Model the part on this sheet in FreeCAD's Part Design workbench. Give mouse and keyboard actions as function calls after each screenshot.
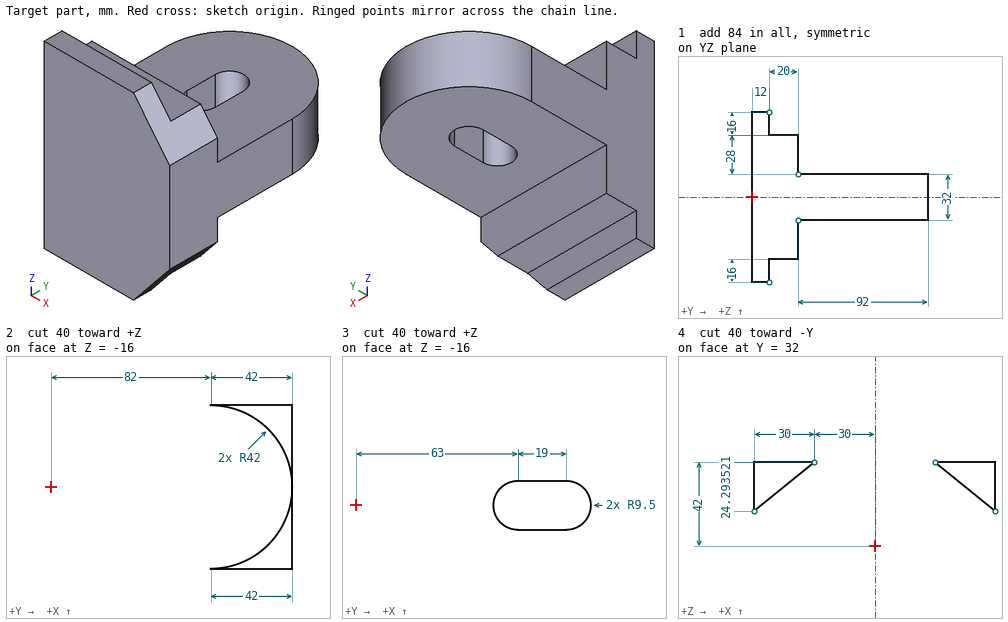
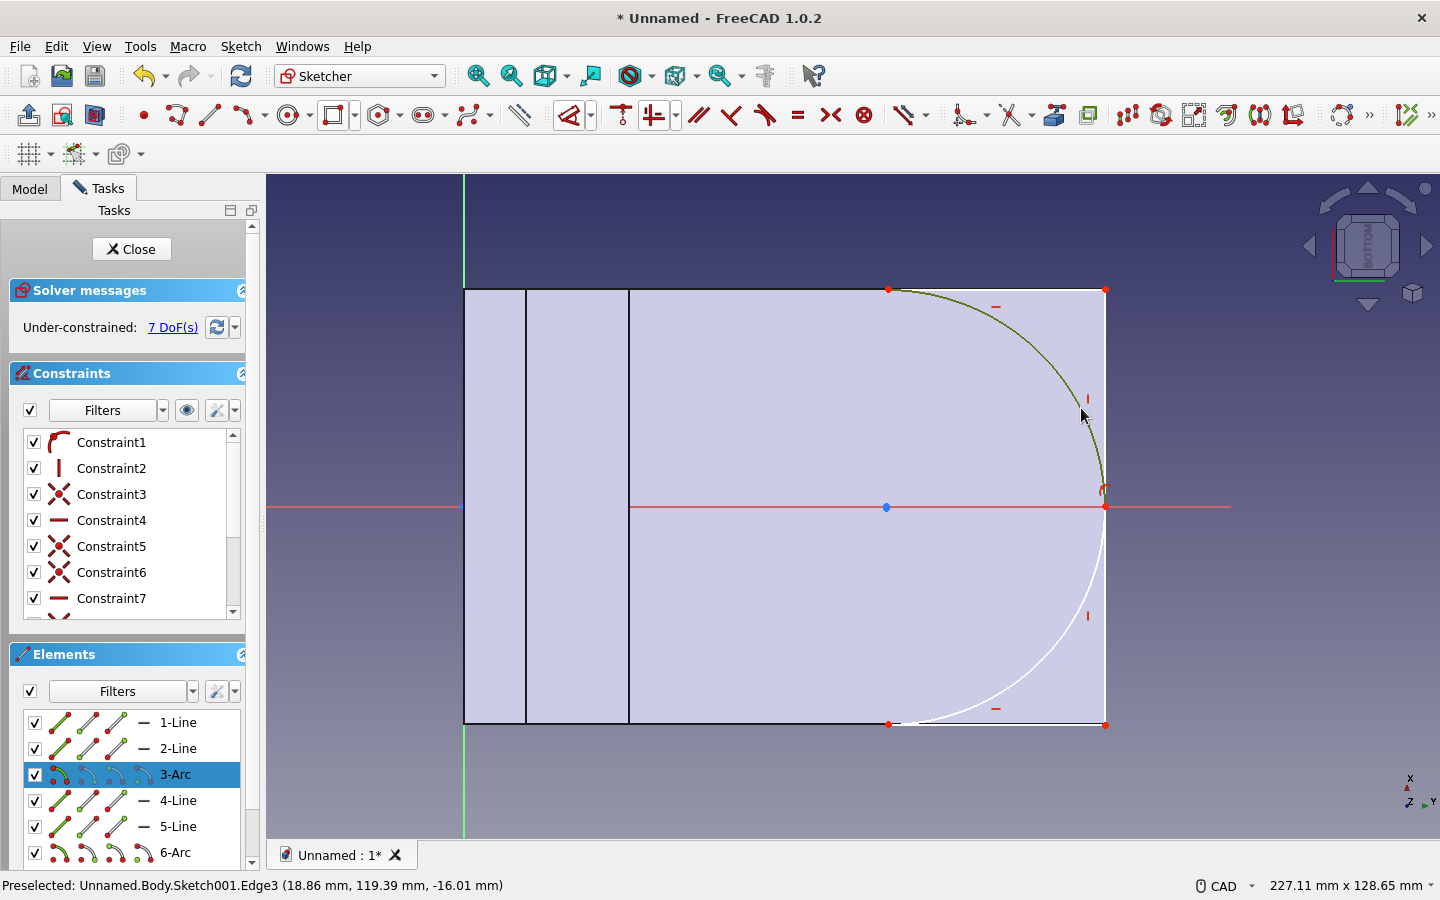
click(987, 701)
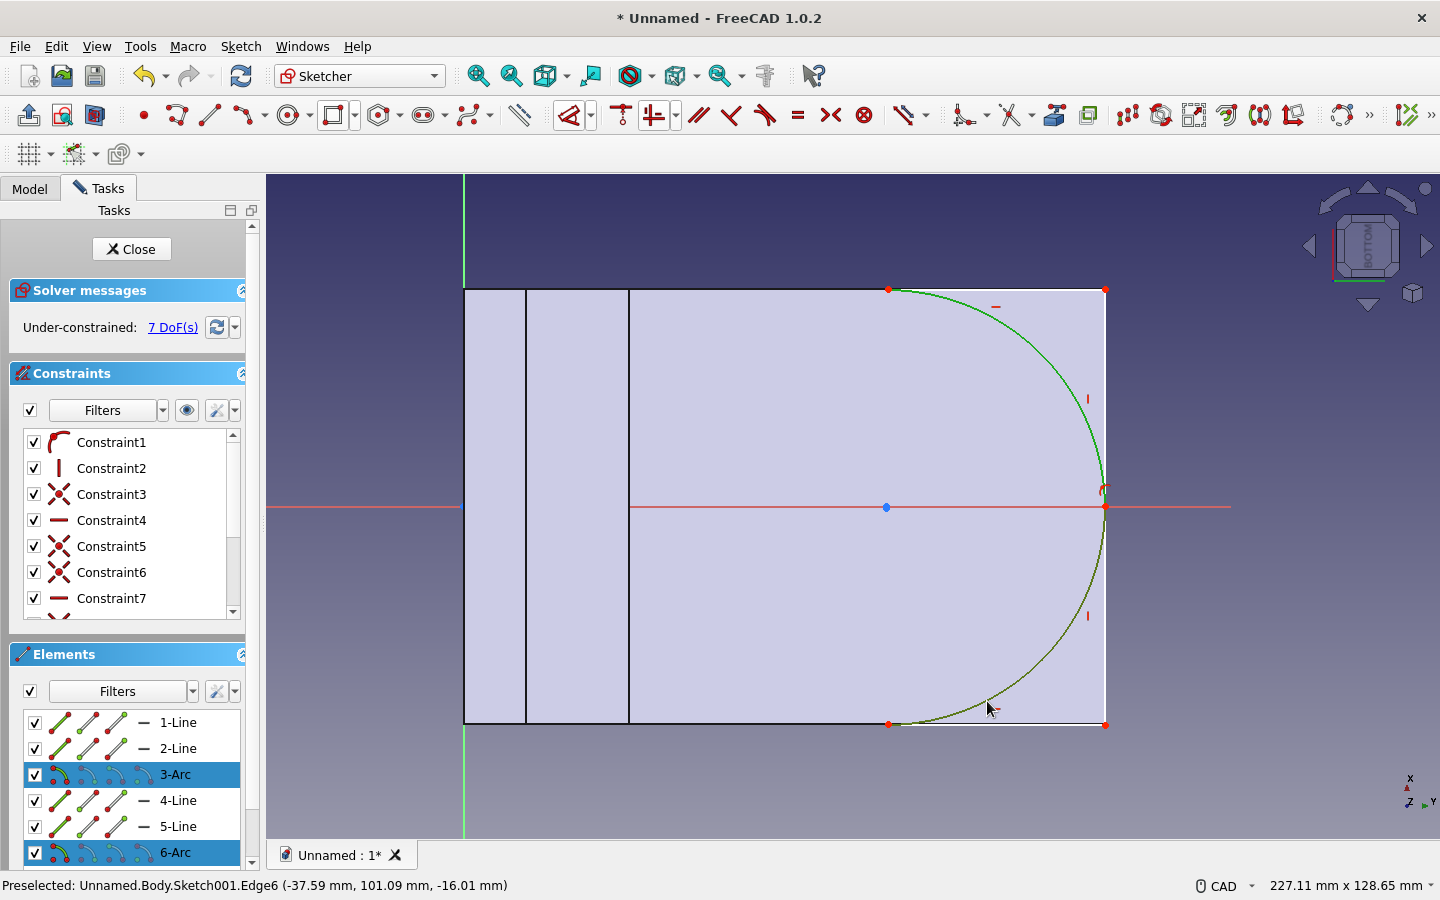
key(c)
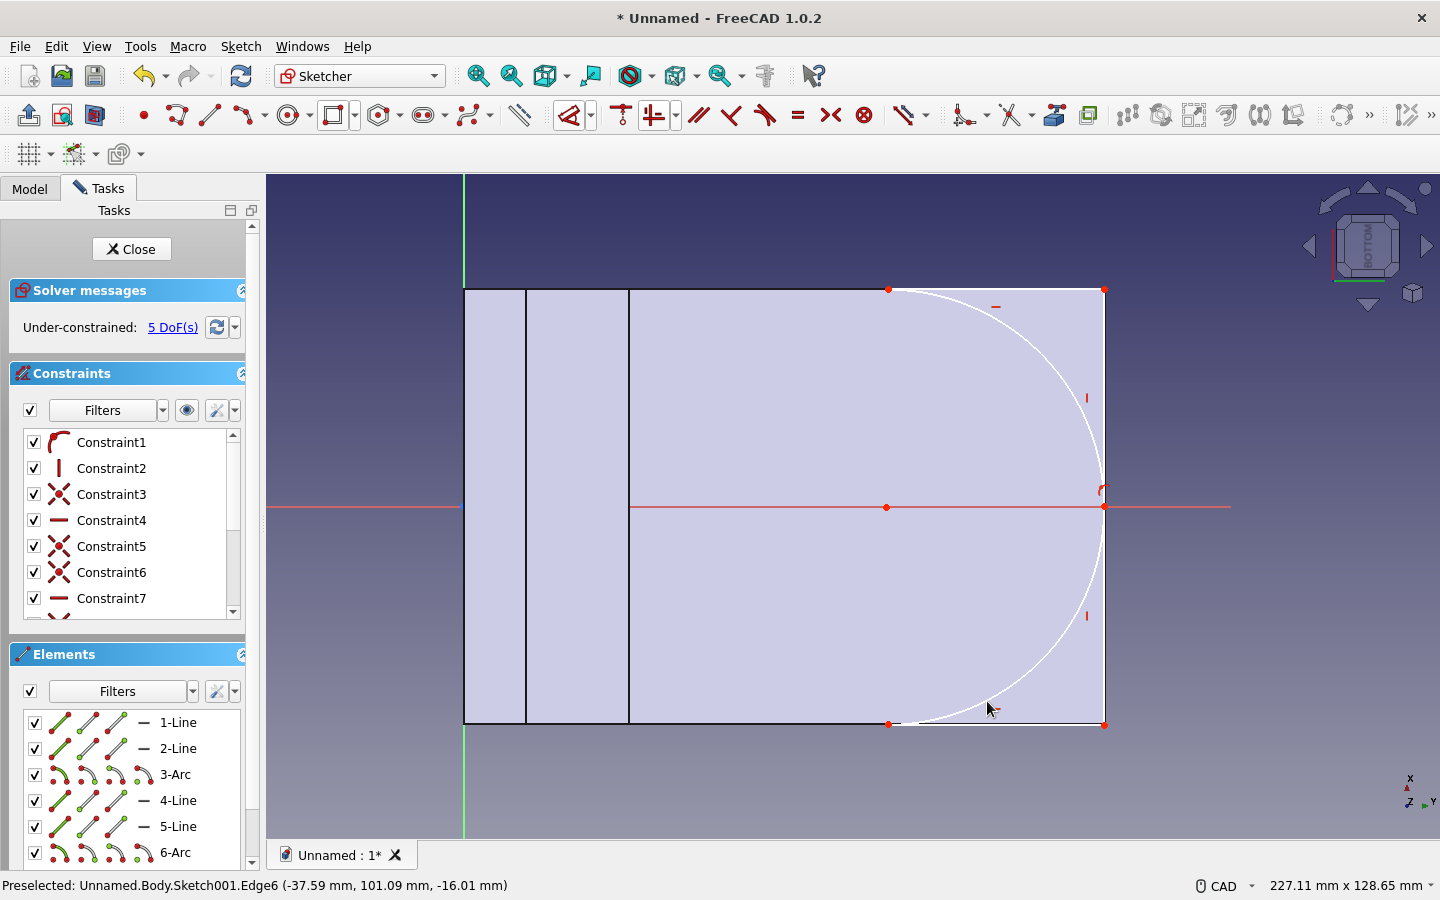
click(886, 507)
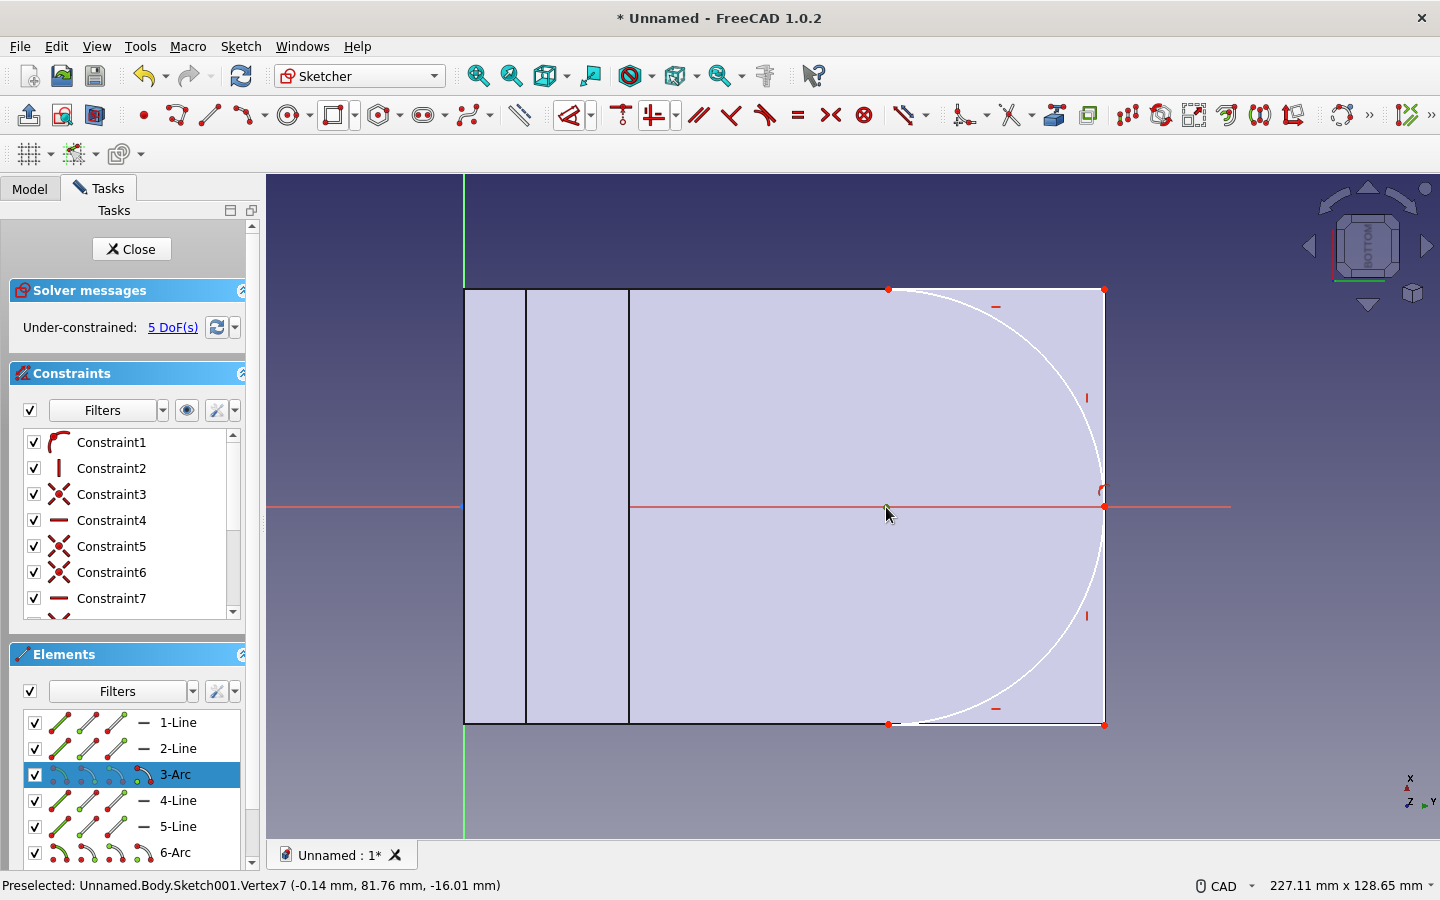
click(364, 506)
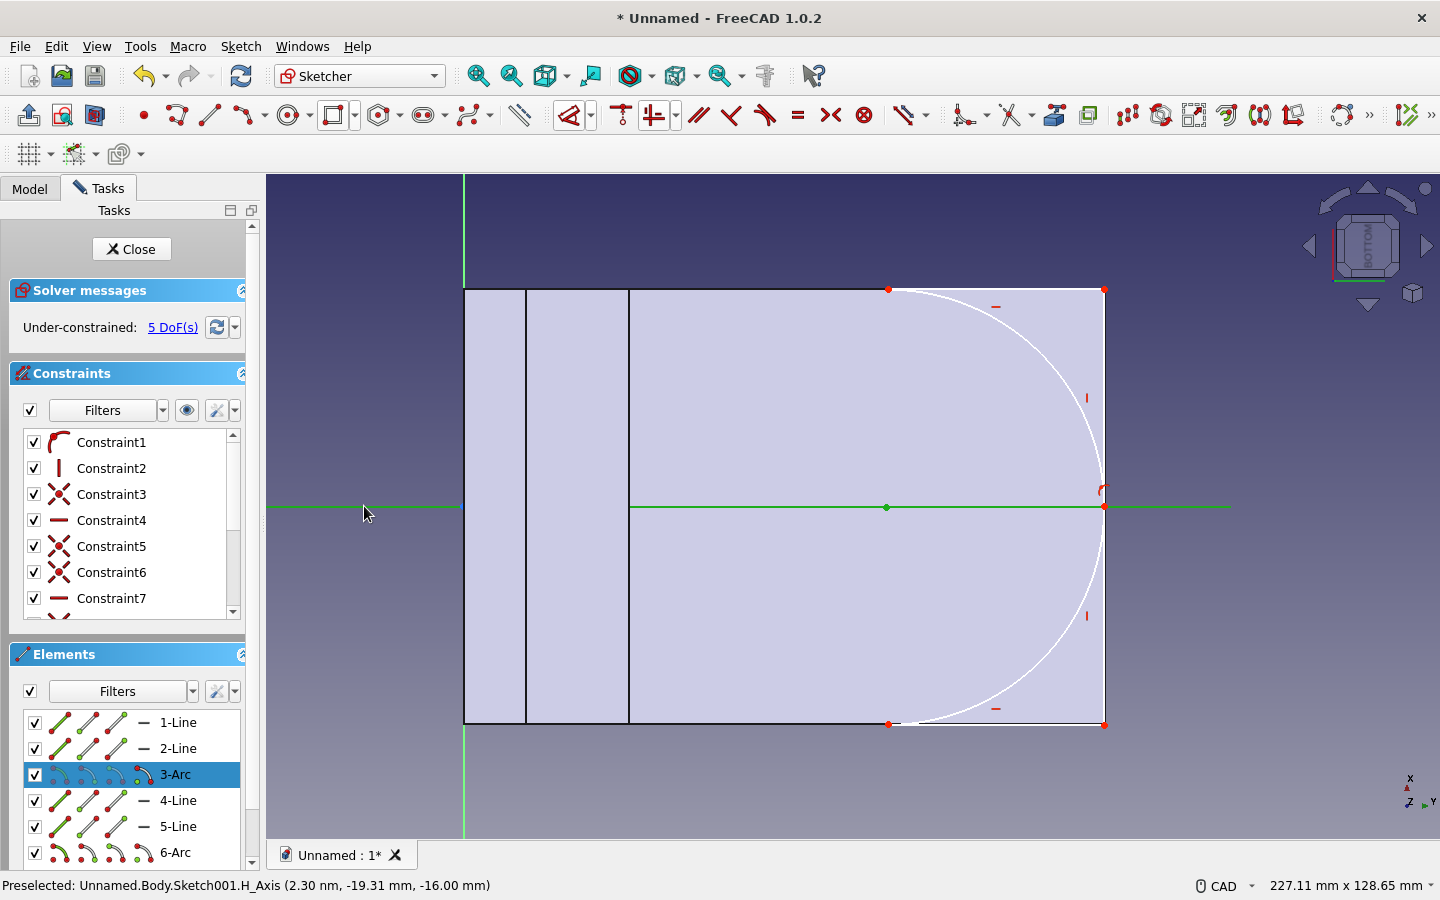
key(c)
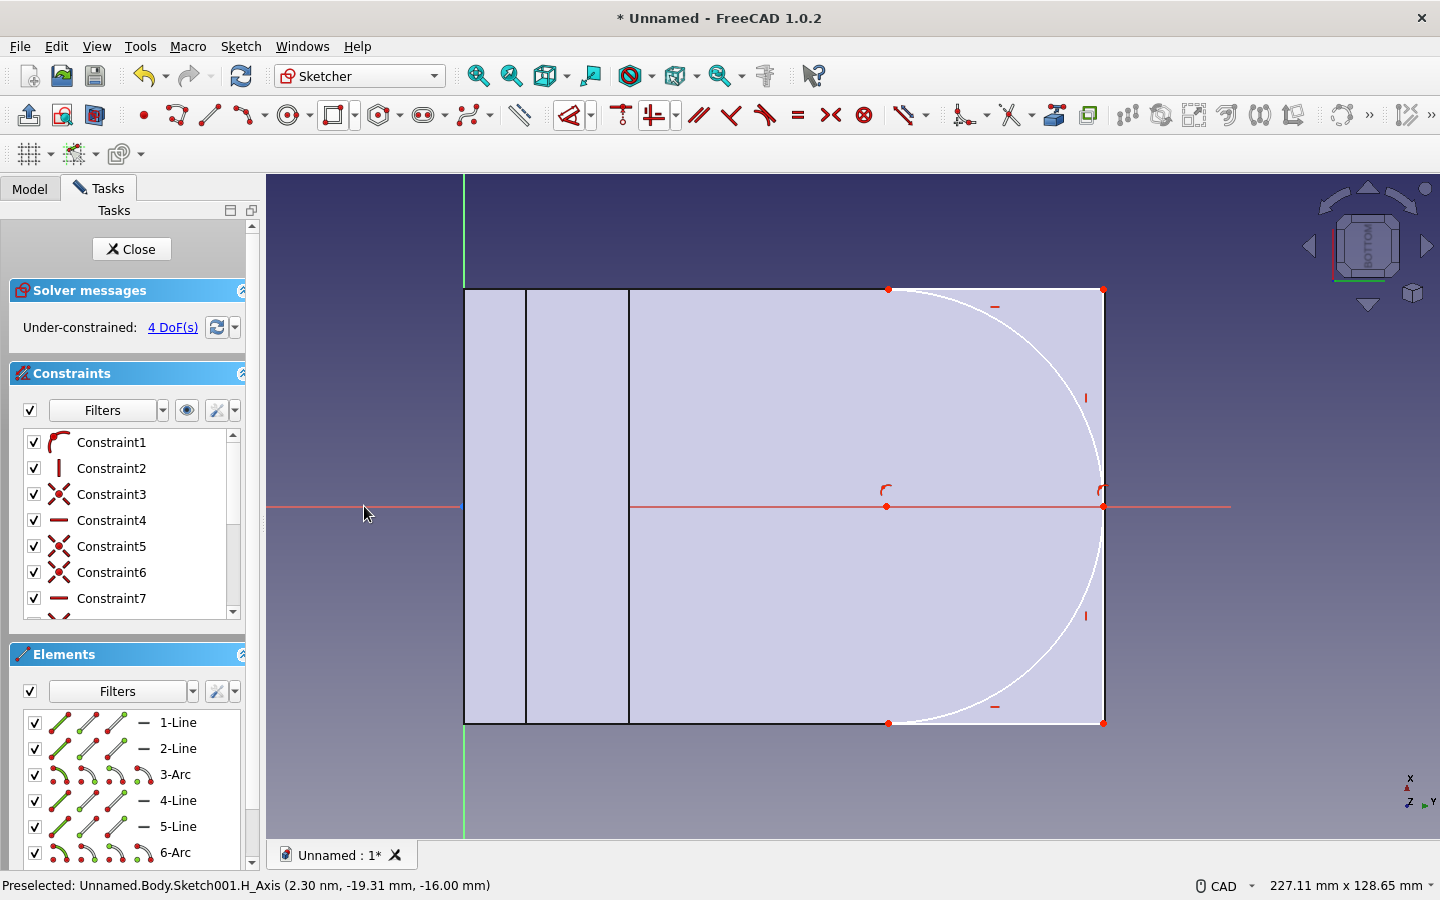
click(1080, 408)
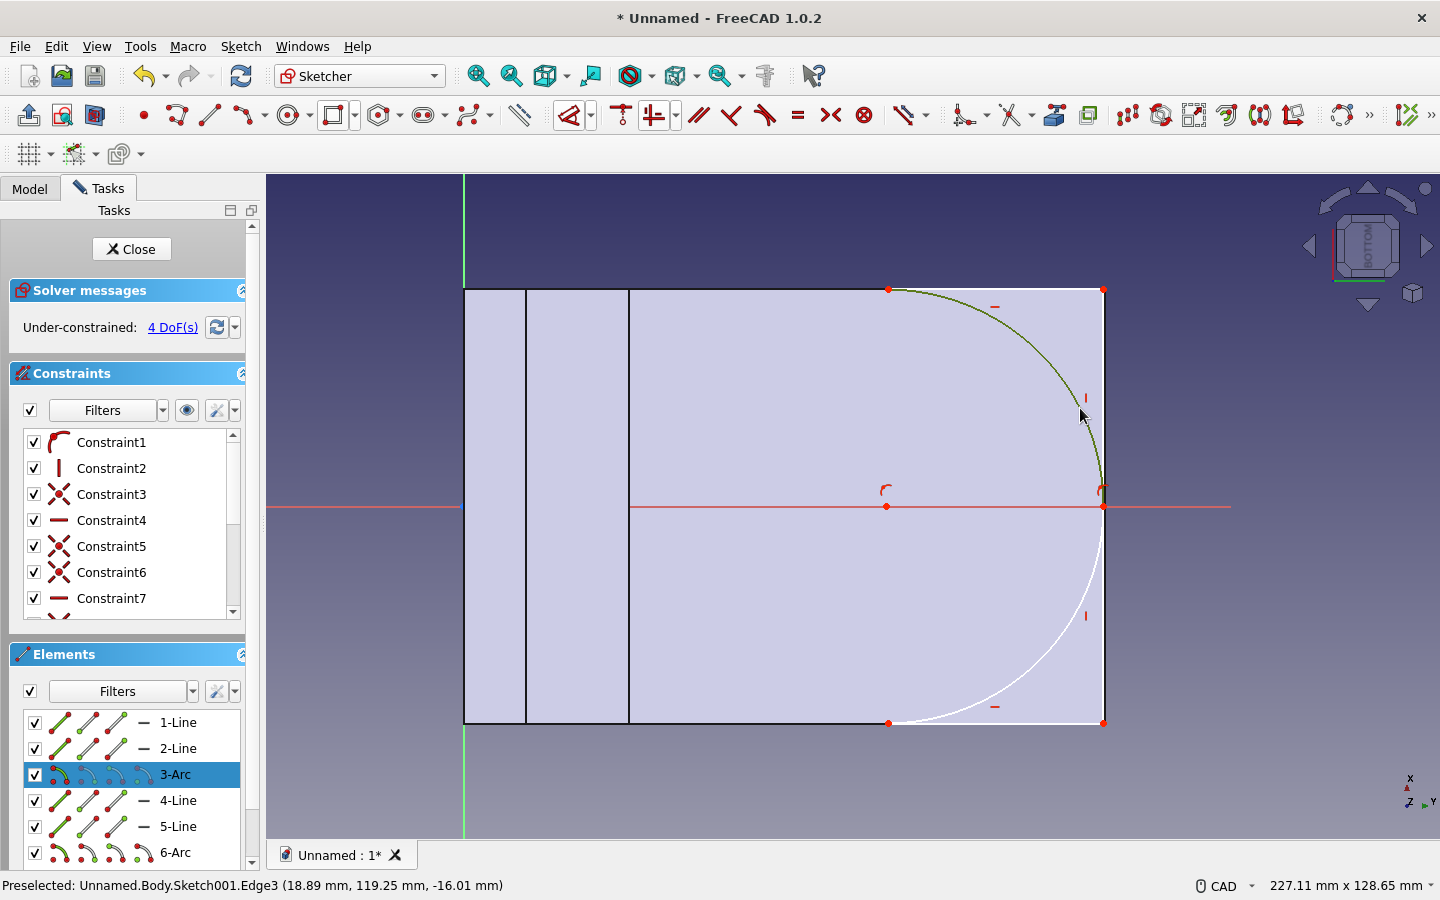
key(k)
key(r)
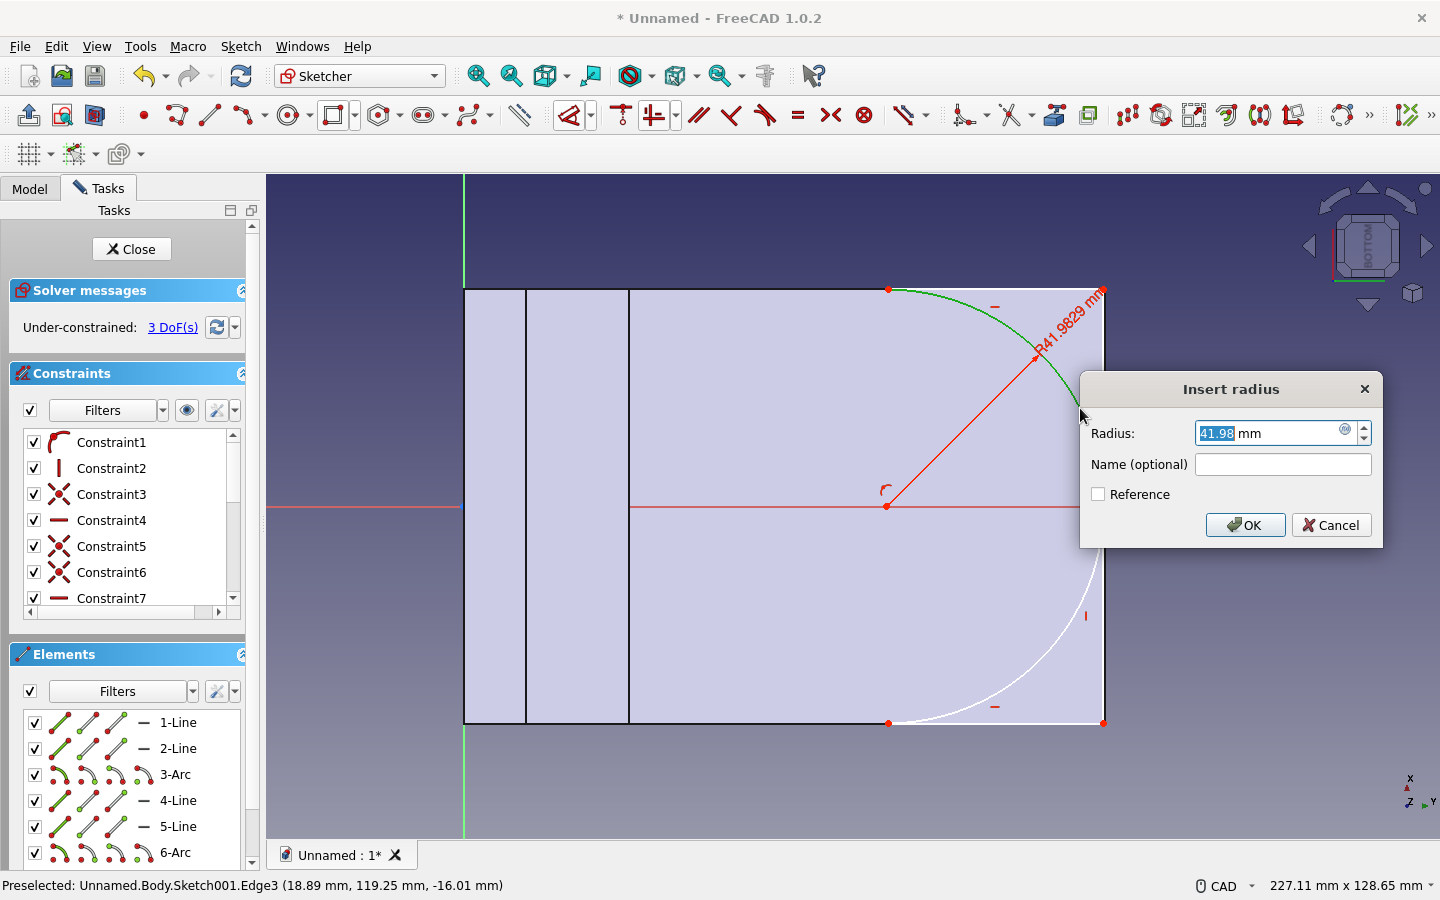
text(42)
key(Return)